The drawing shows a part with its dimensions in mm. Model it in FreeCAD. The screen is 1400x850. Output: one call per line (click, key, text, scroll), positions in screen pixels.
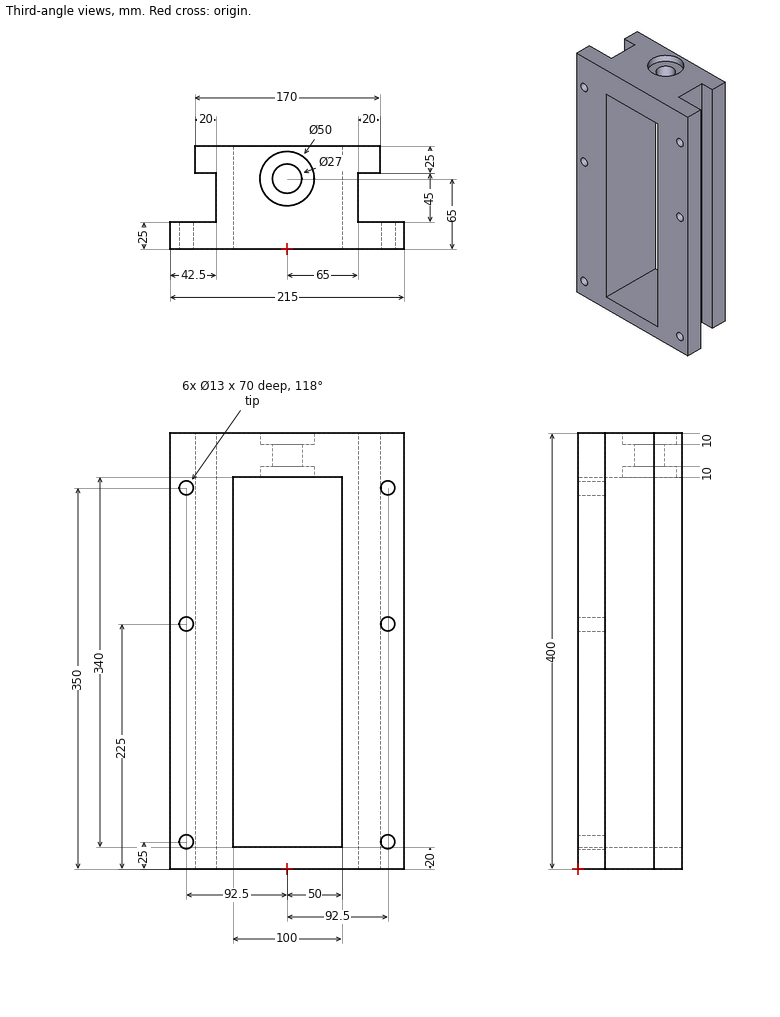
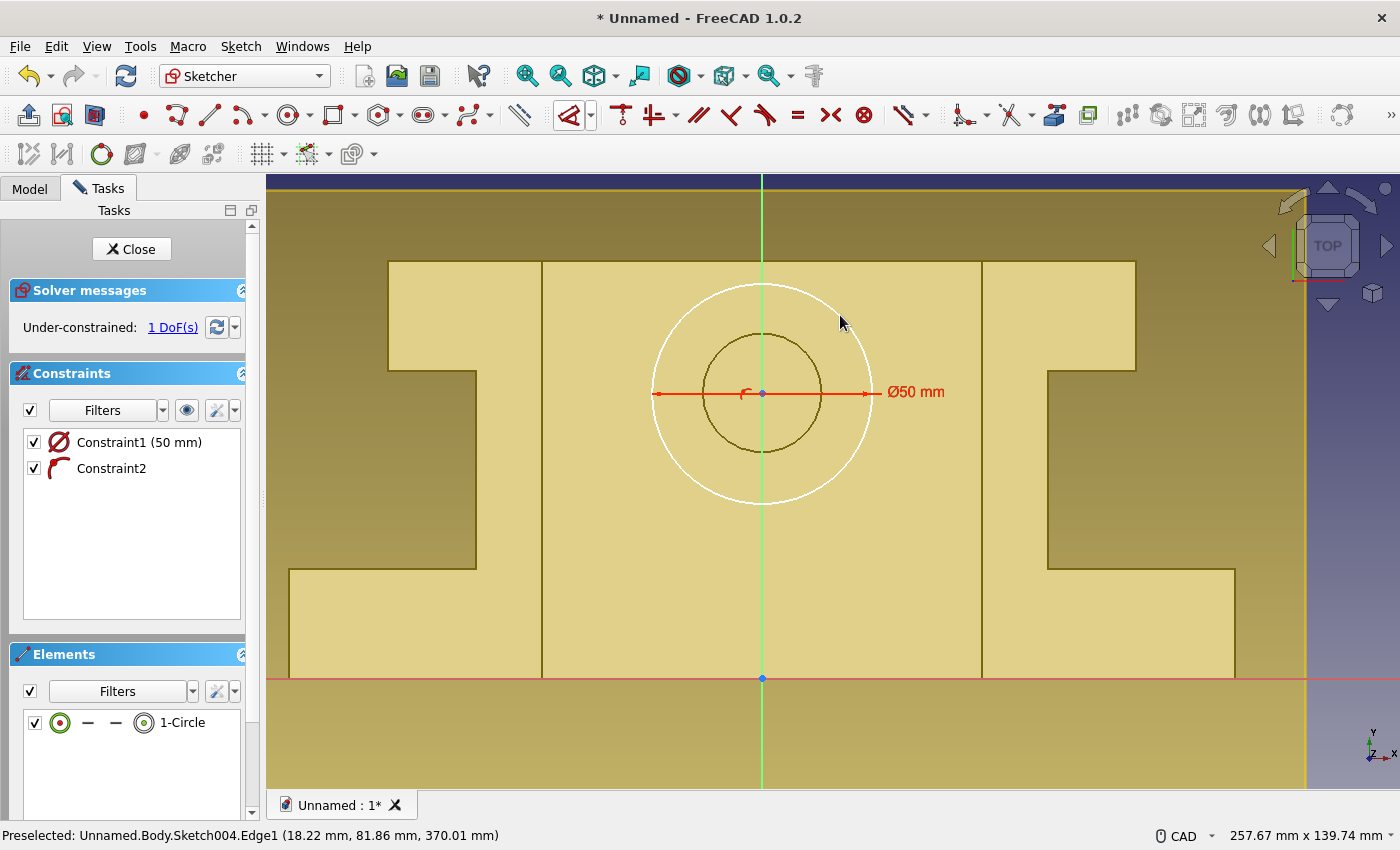
click(762, 394)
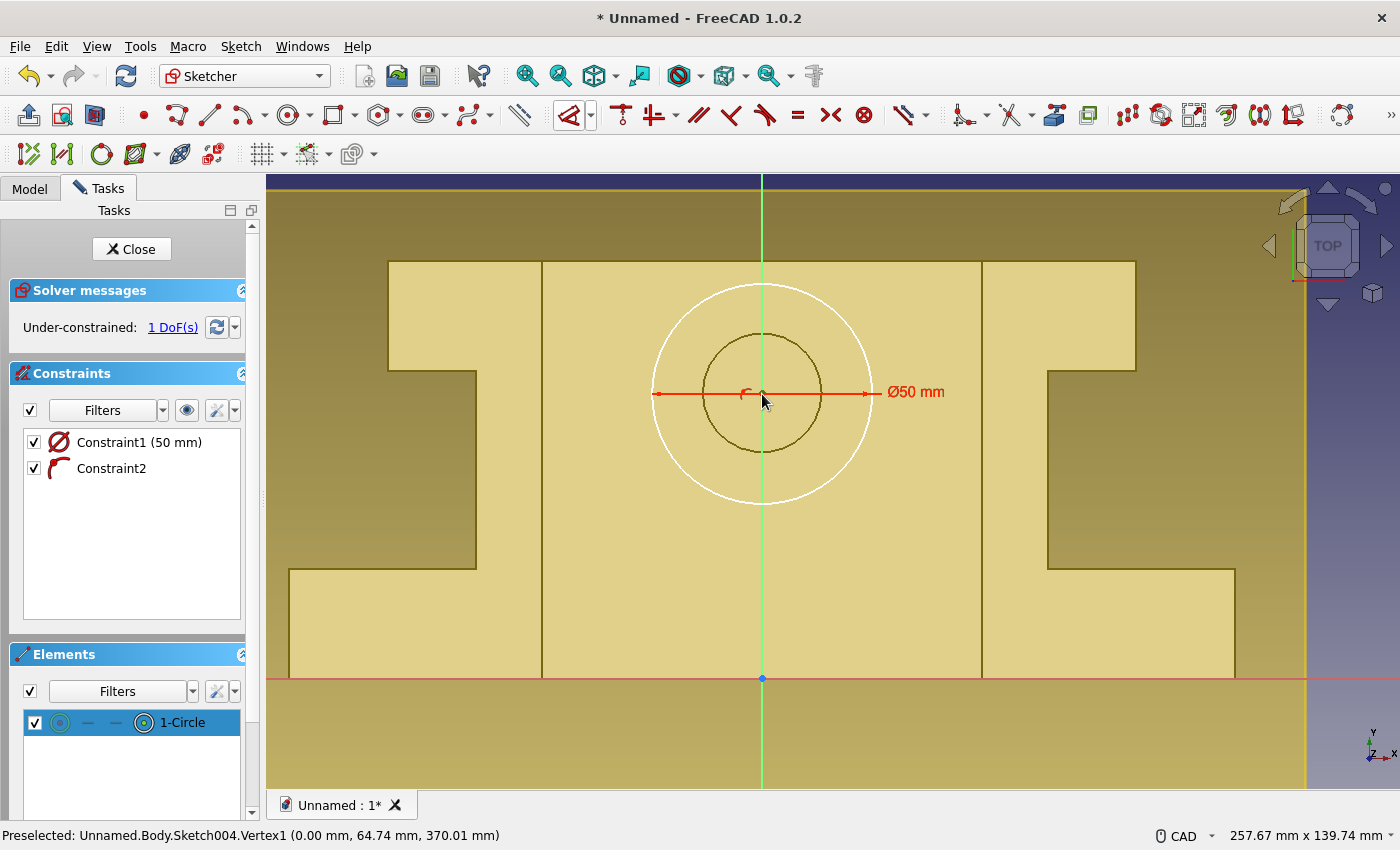
key(i)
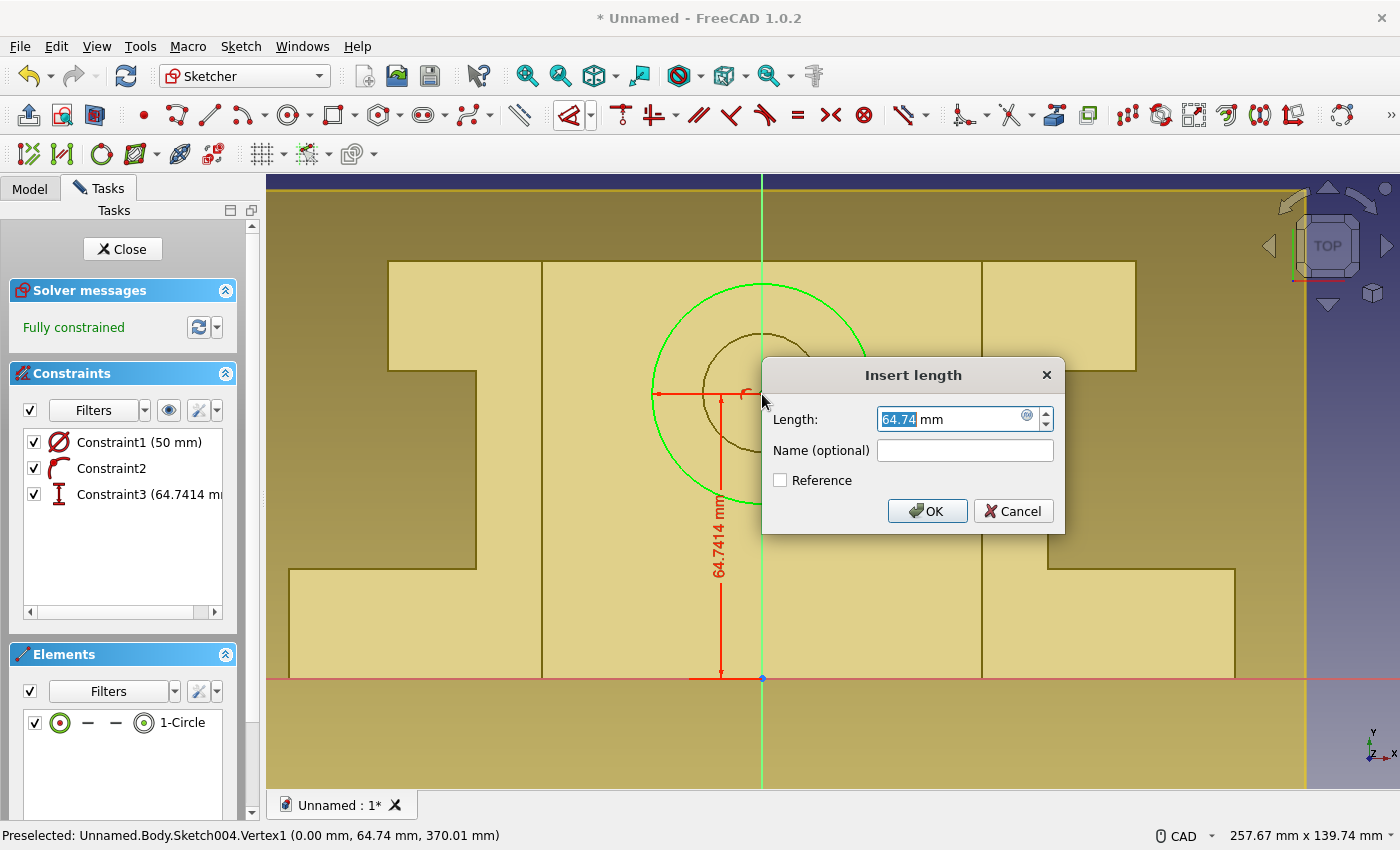
text(65)
key(Return)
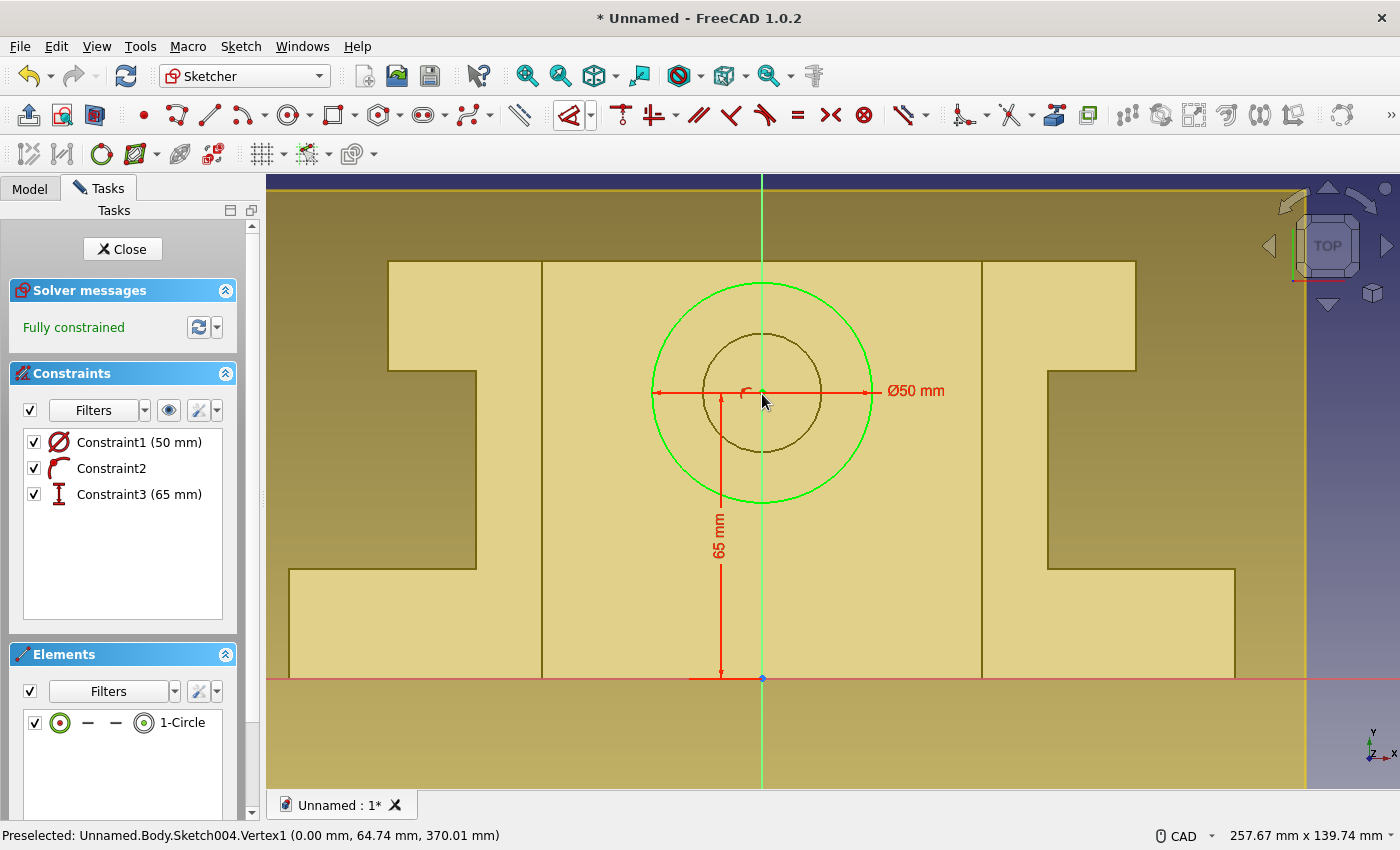
click(123, 249)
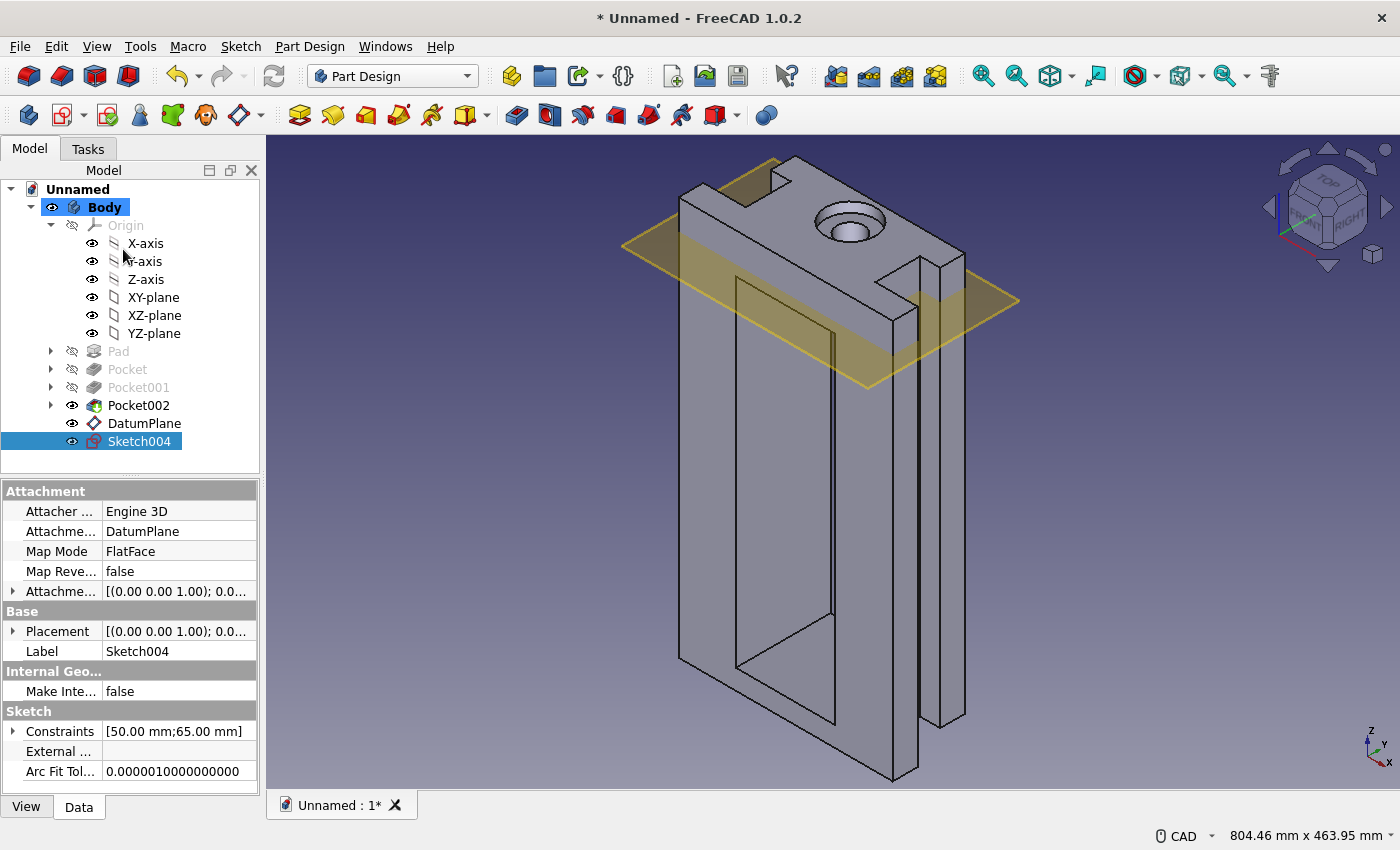
click(517, 116)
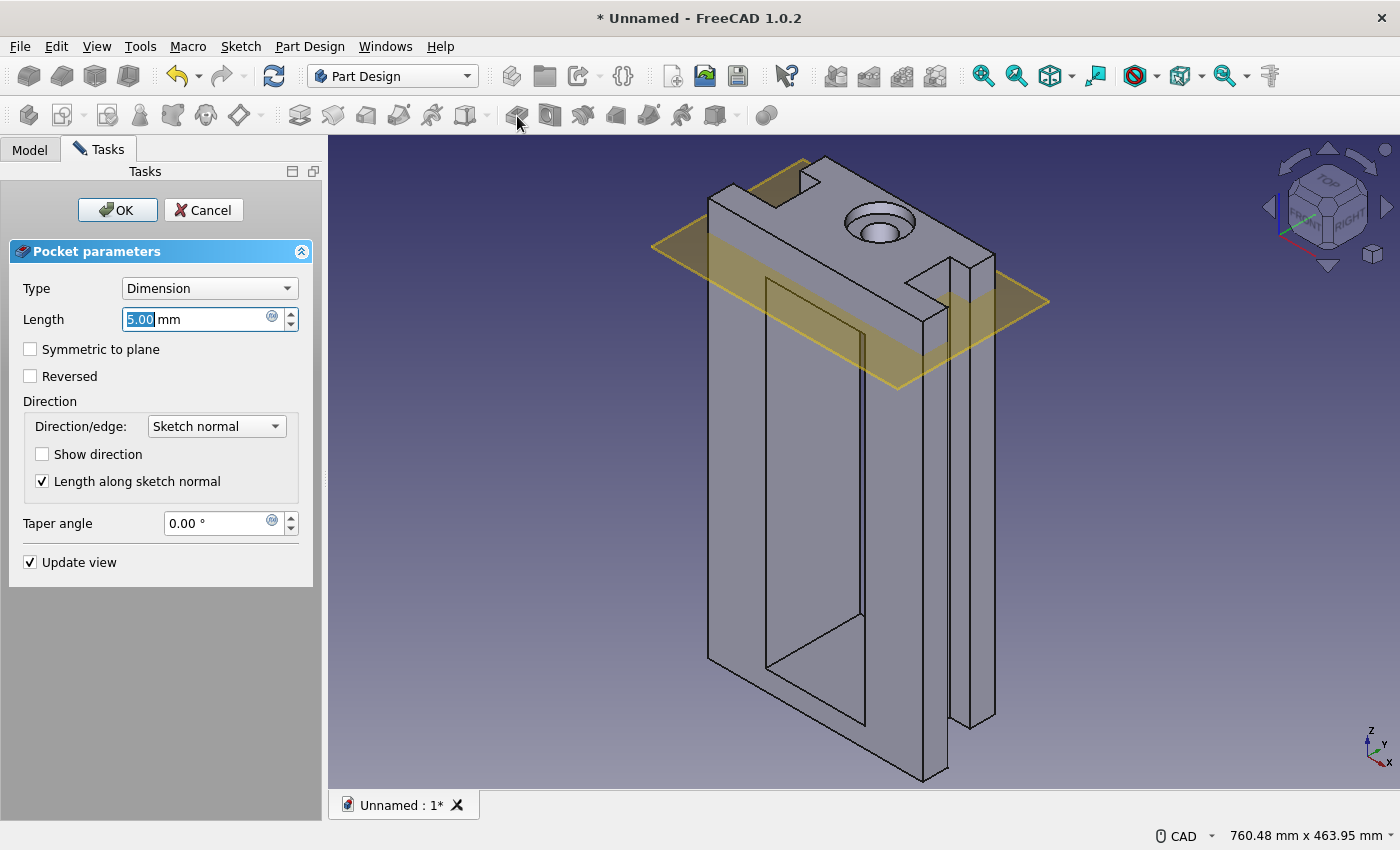
text(10)
key(Tab)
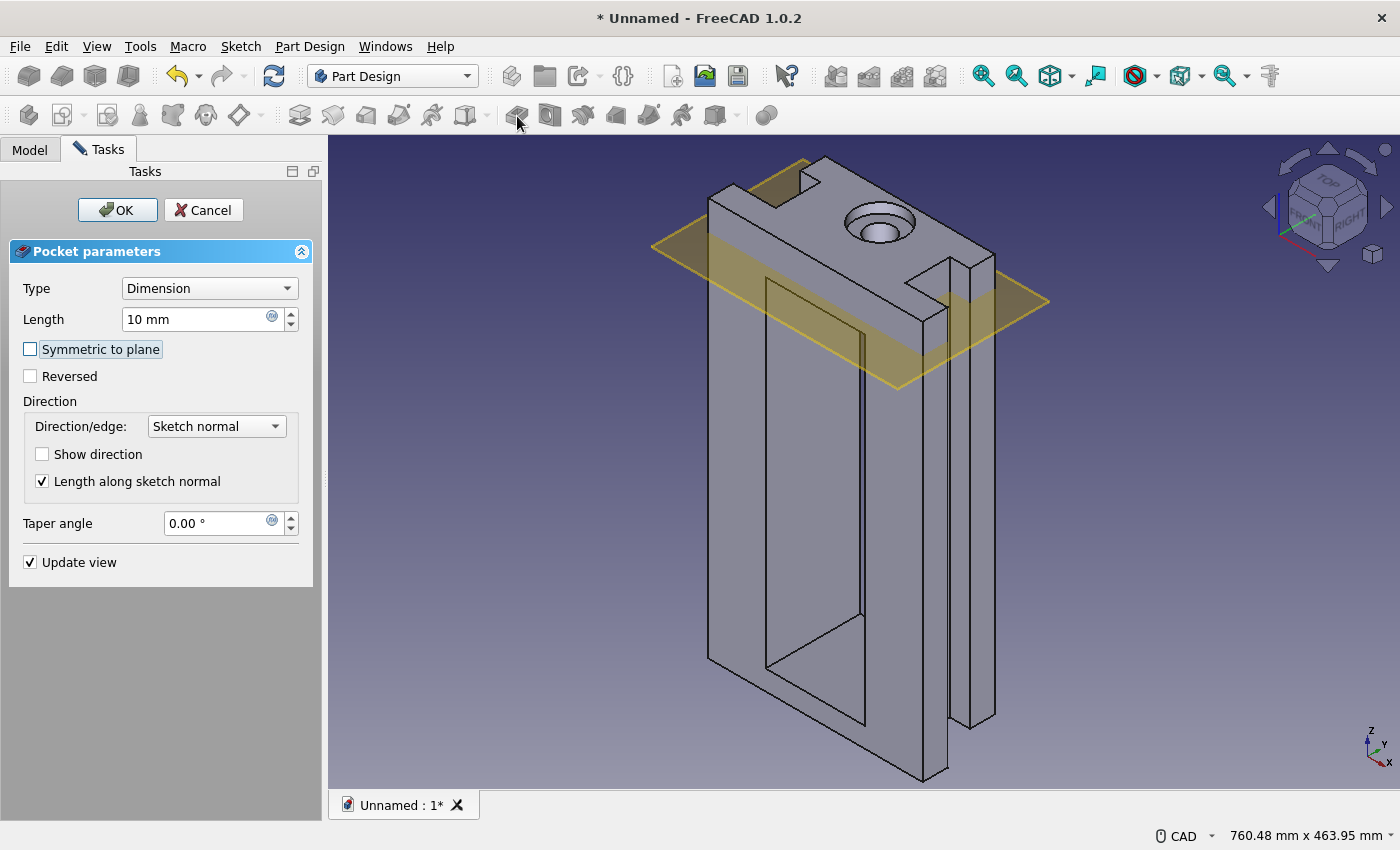
click(118, 210)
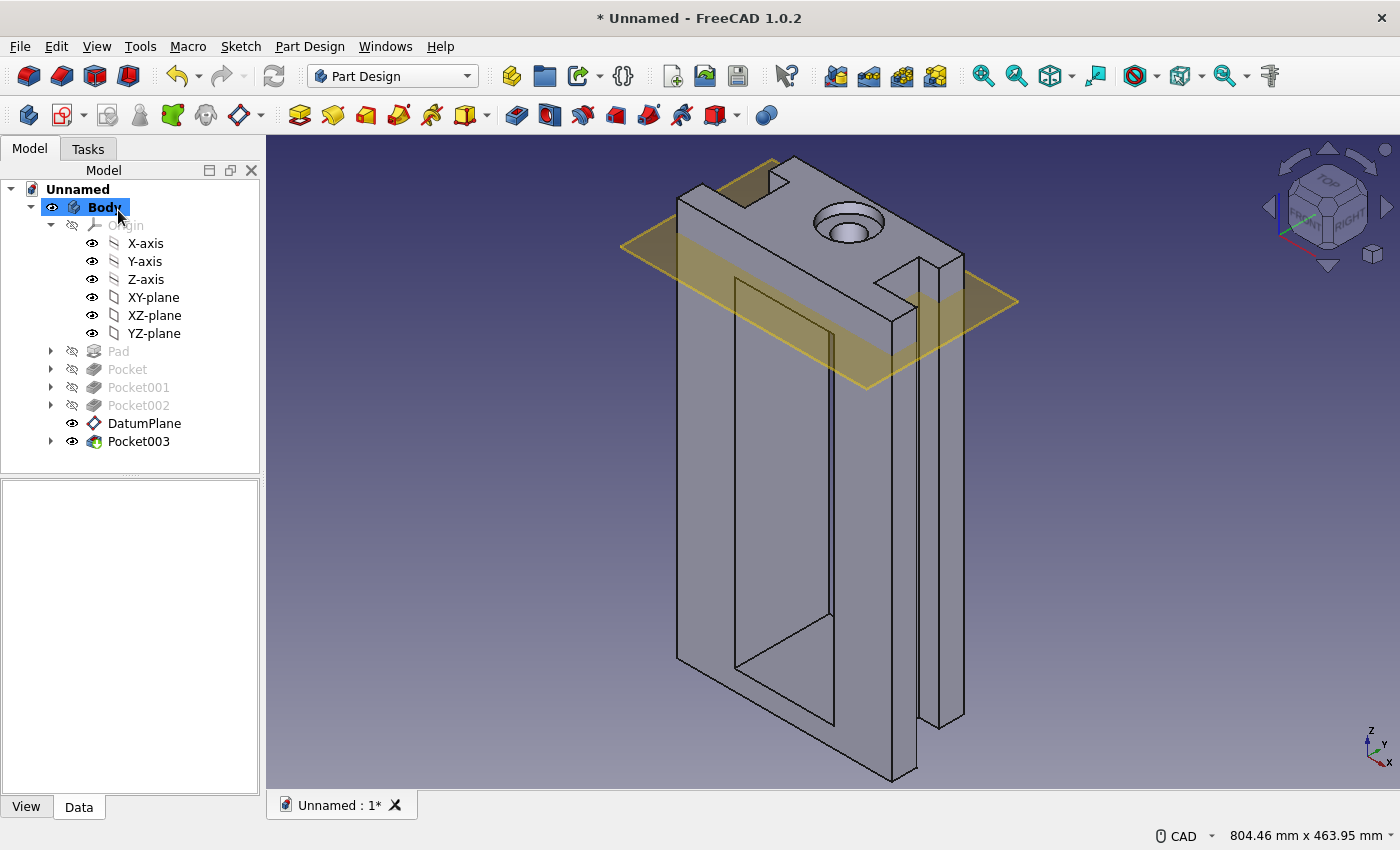
click(117, 423)
key(space)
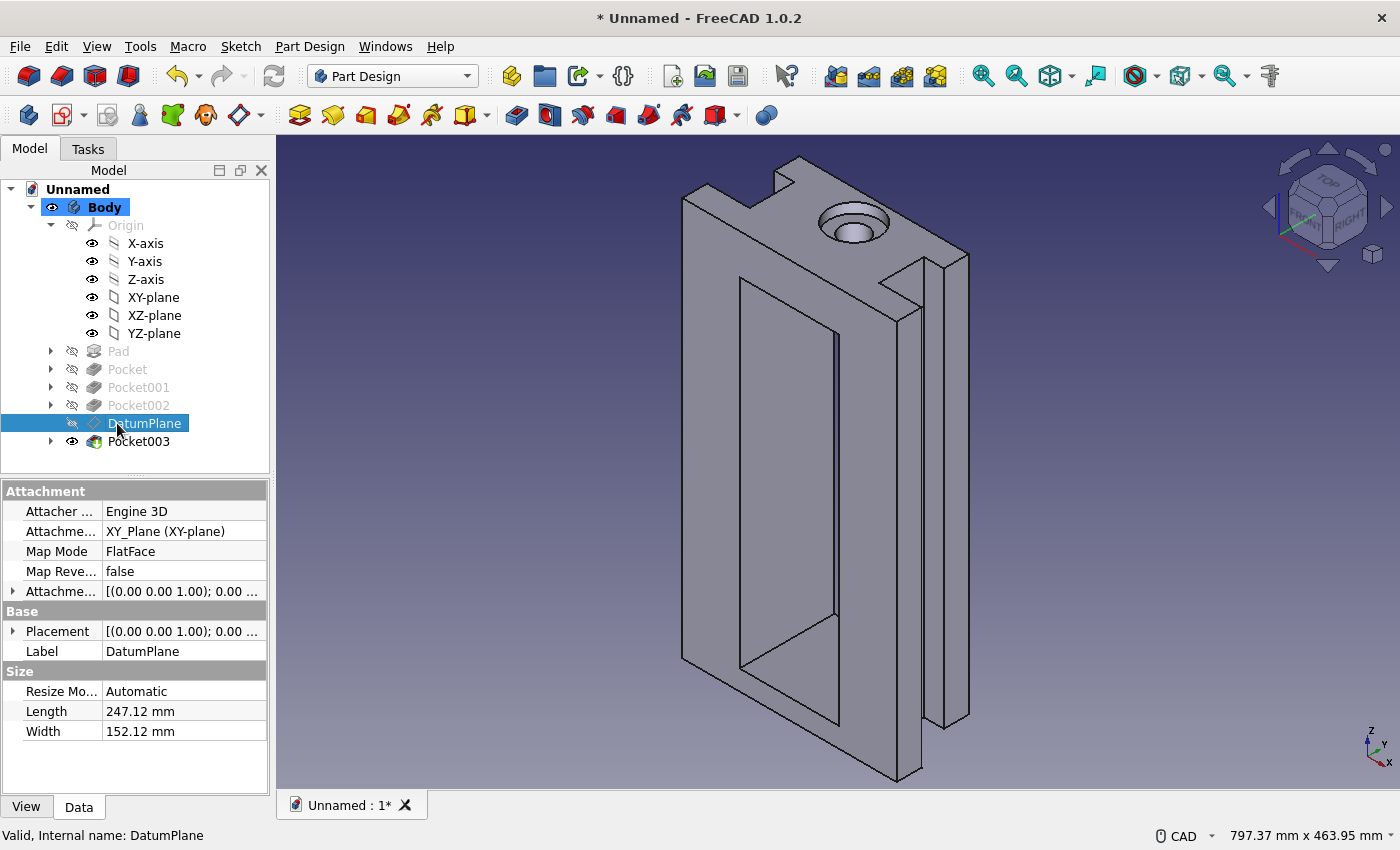
key(4)